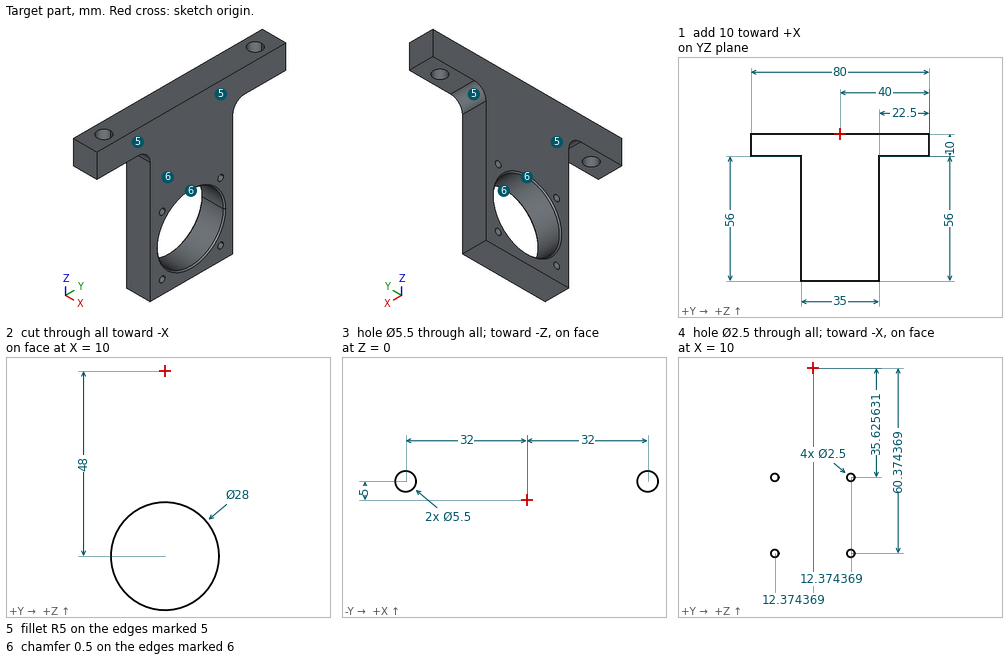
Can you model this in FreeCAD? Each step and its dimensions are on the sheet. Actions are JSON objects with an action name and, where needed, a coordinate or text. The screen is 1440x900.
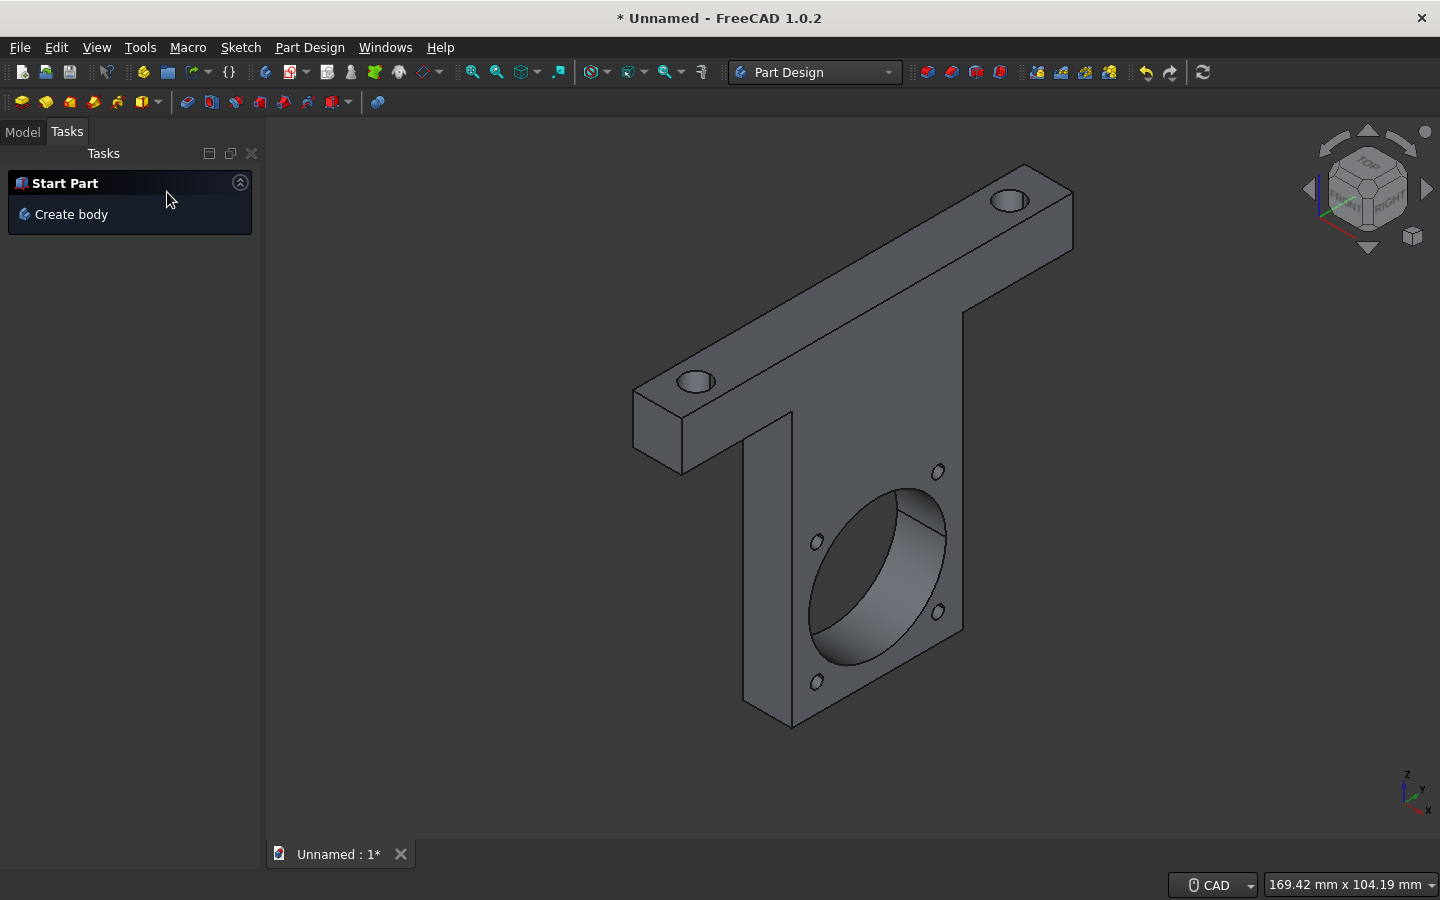
{"action": "key", "text": "2"}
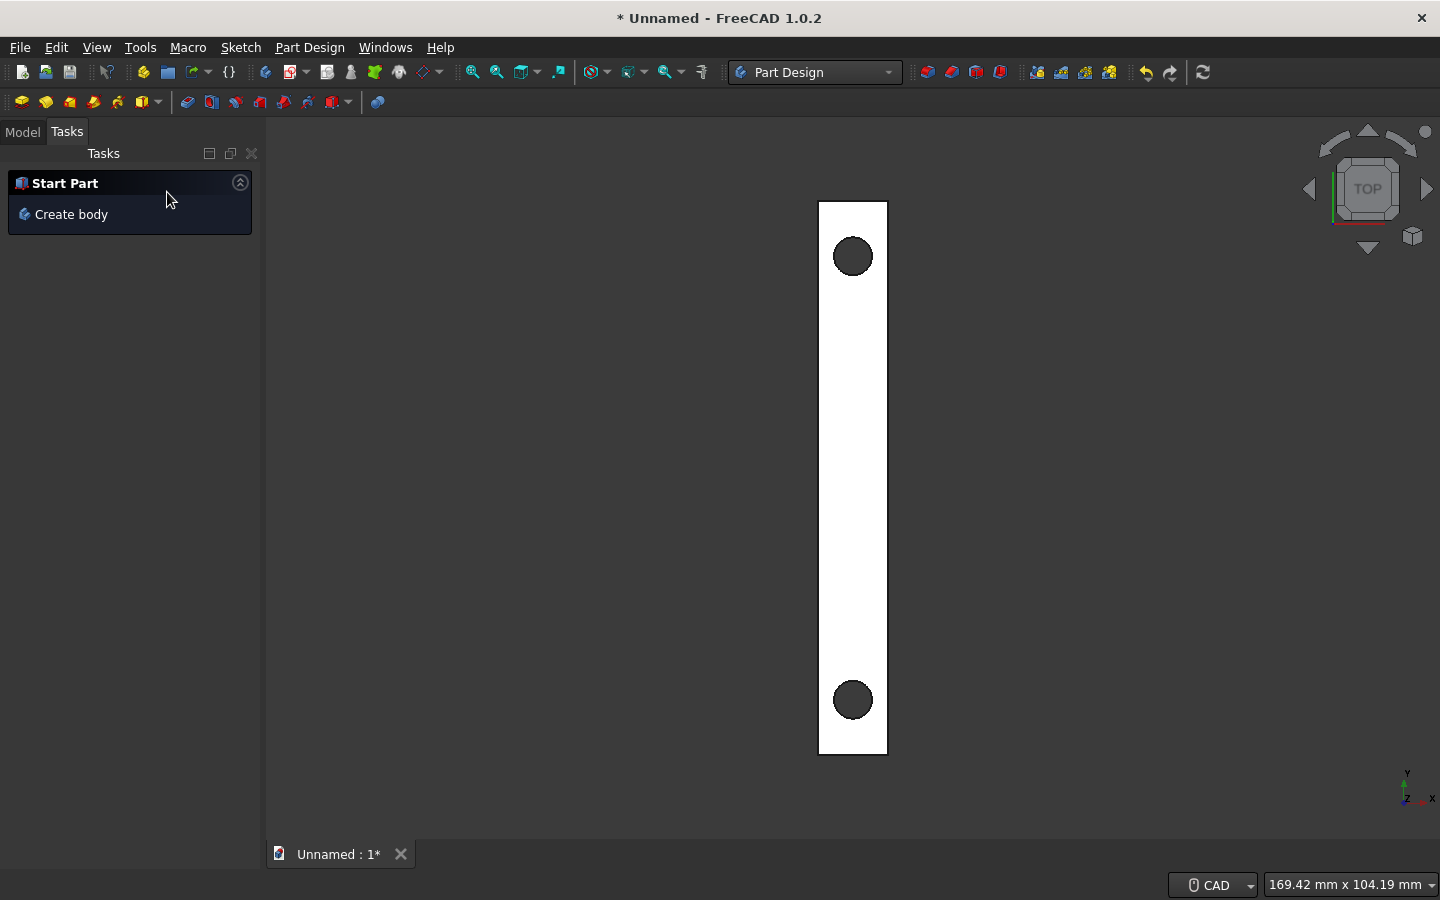
{"action": "key", "text": "1"}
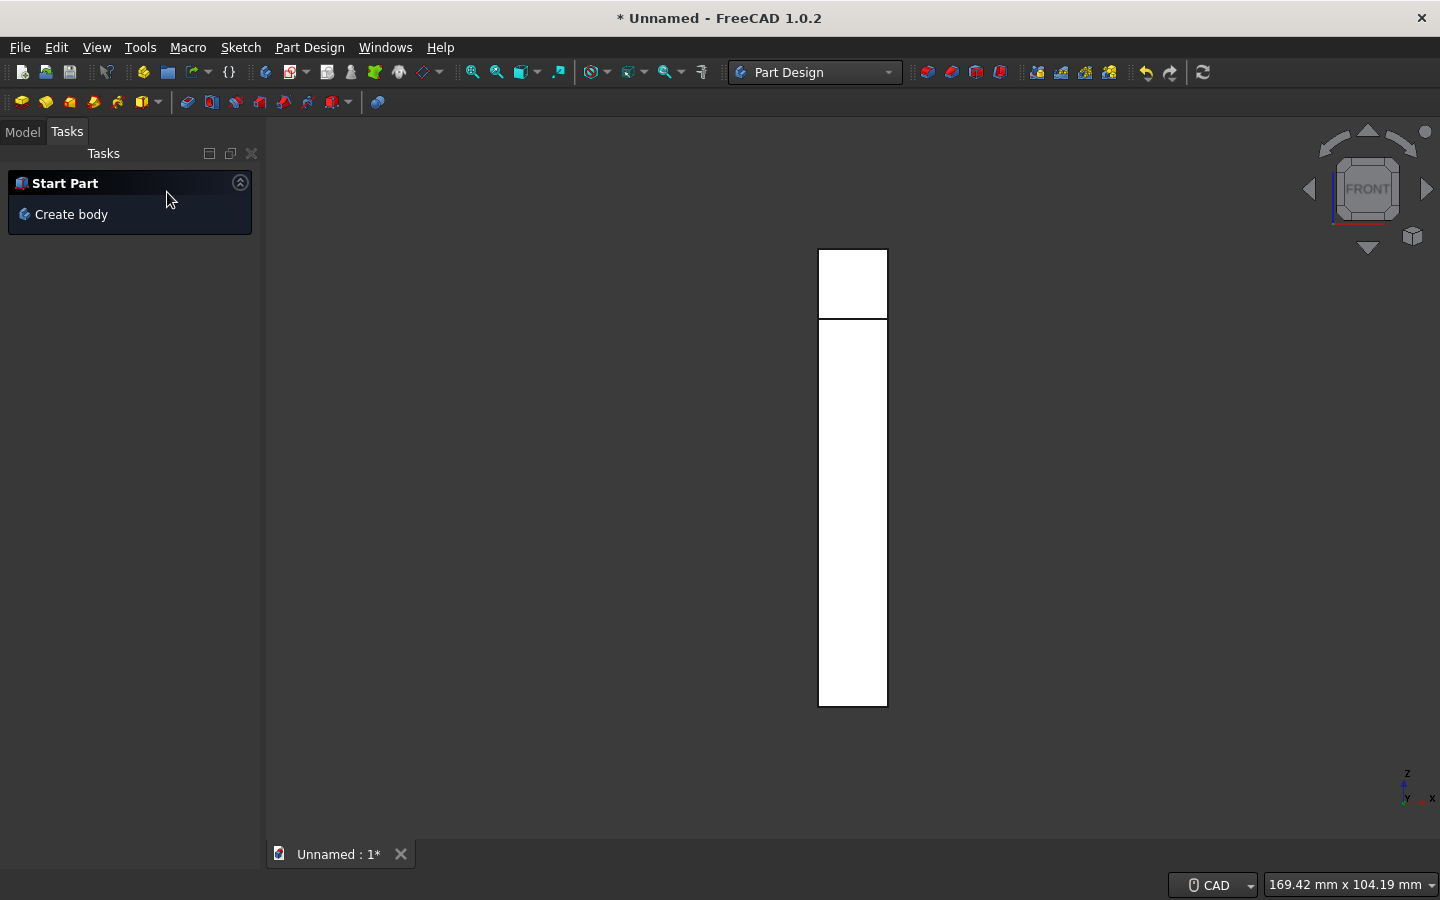
{"action": "key", "text": "3"}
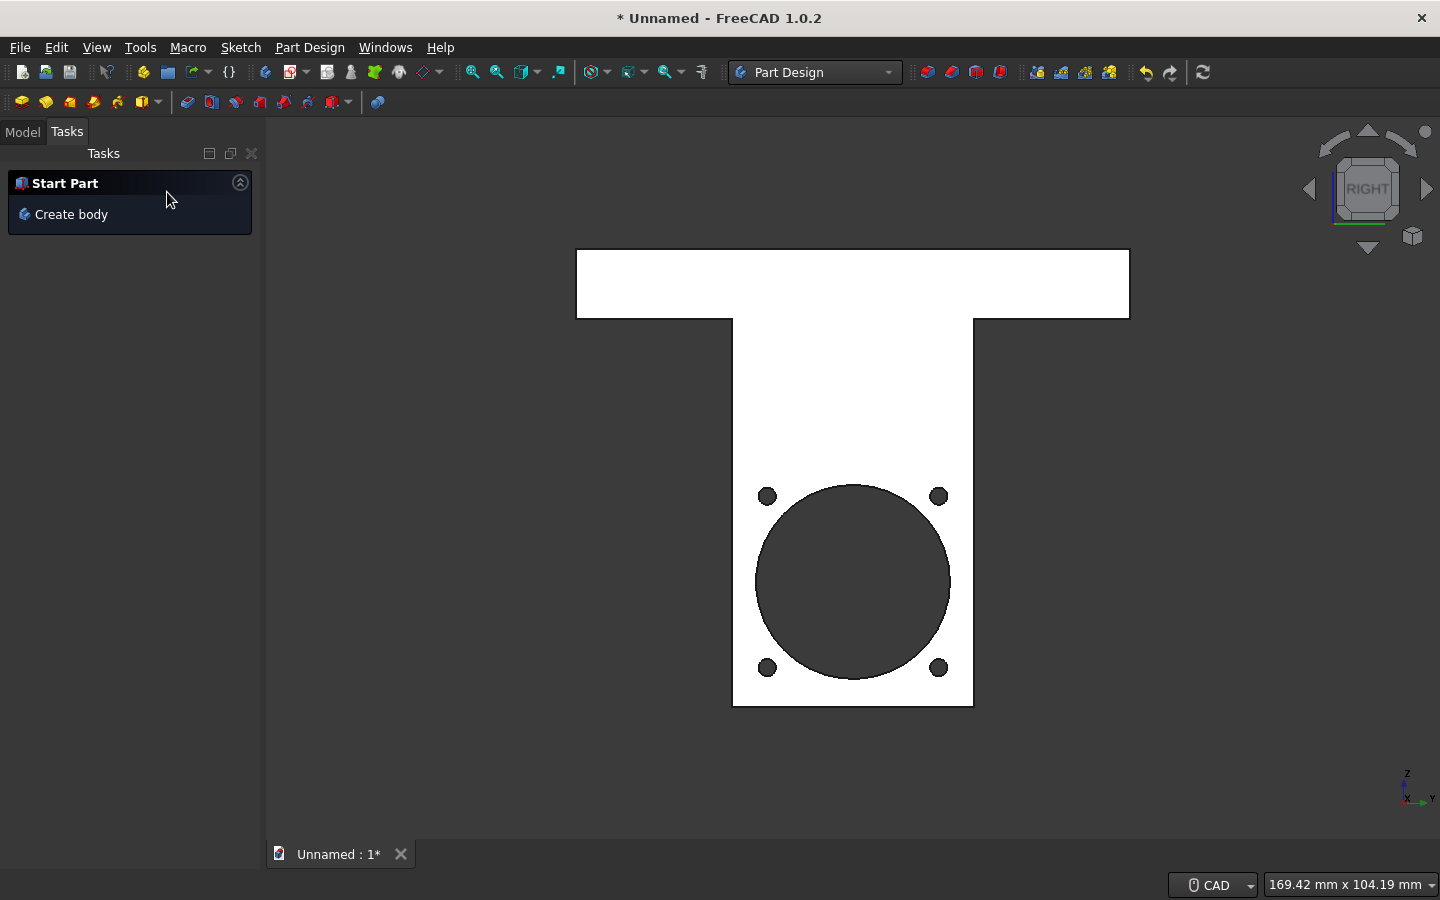
{"action": "key", "text": "5"}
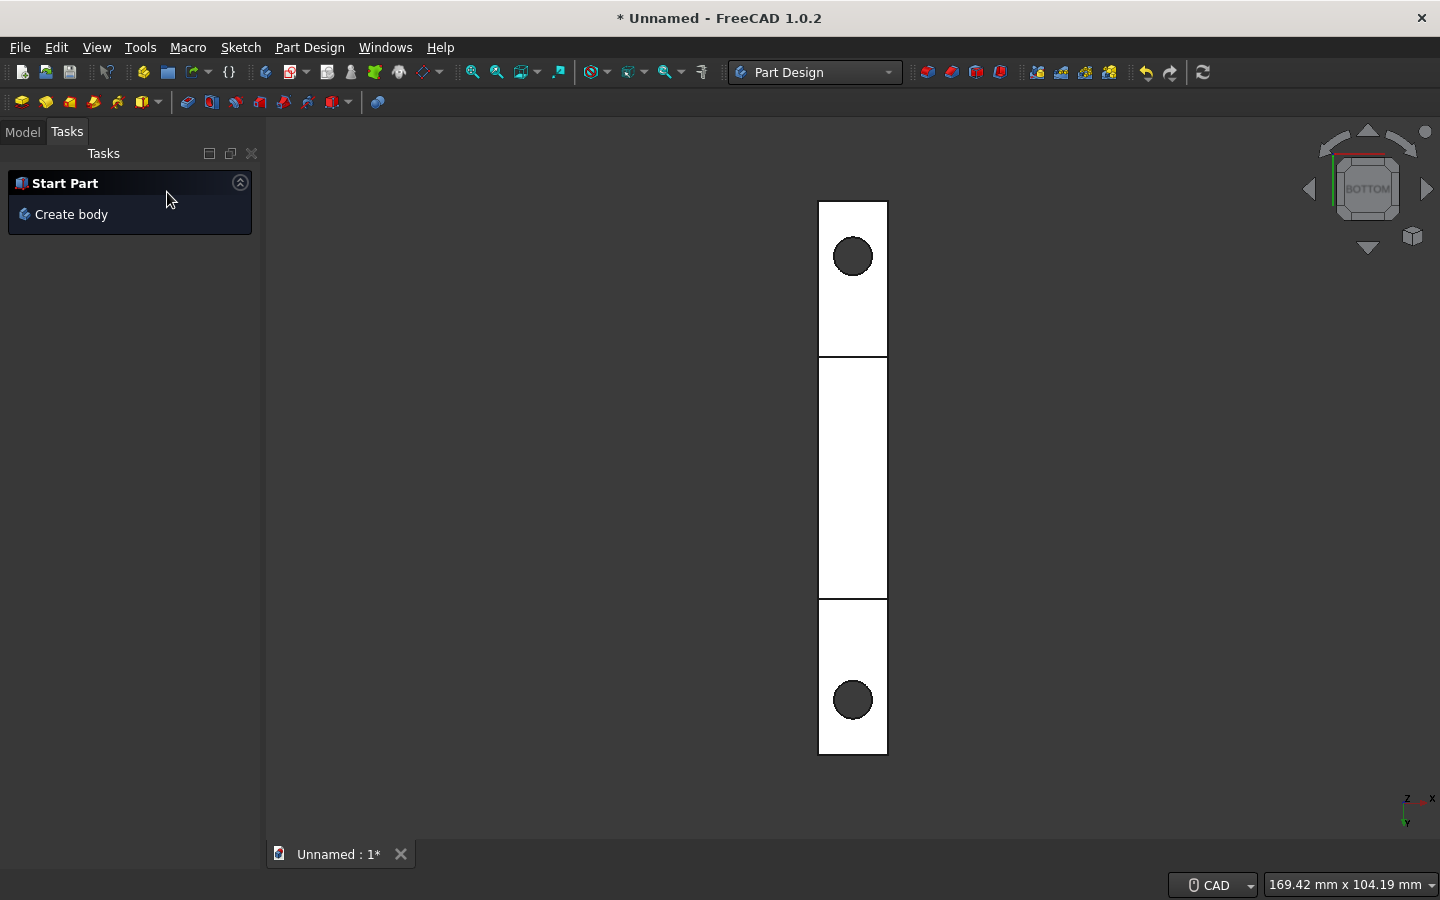
{"action": "key", "text": "4"}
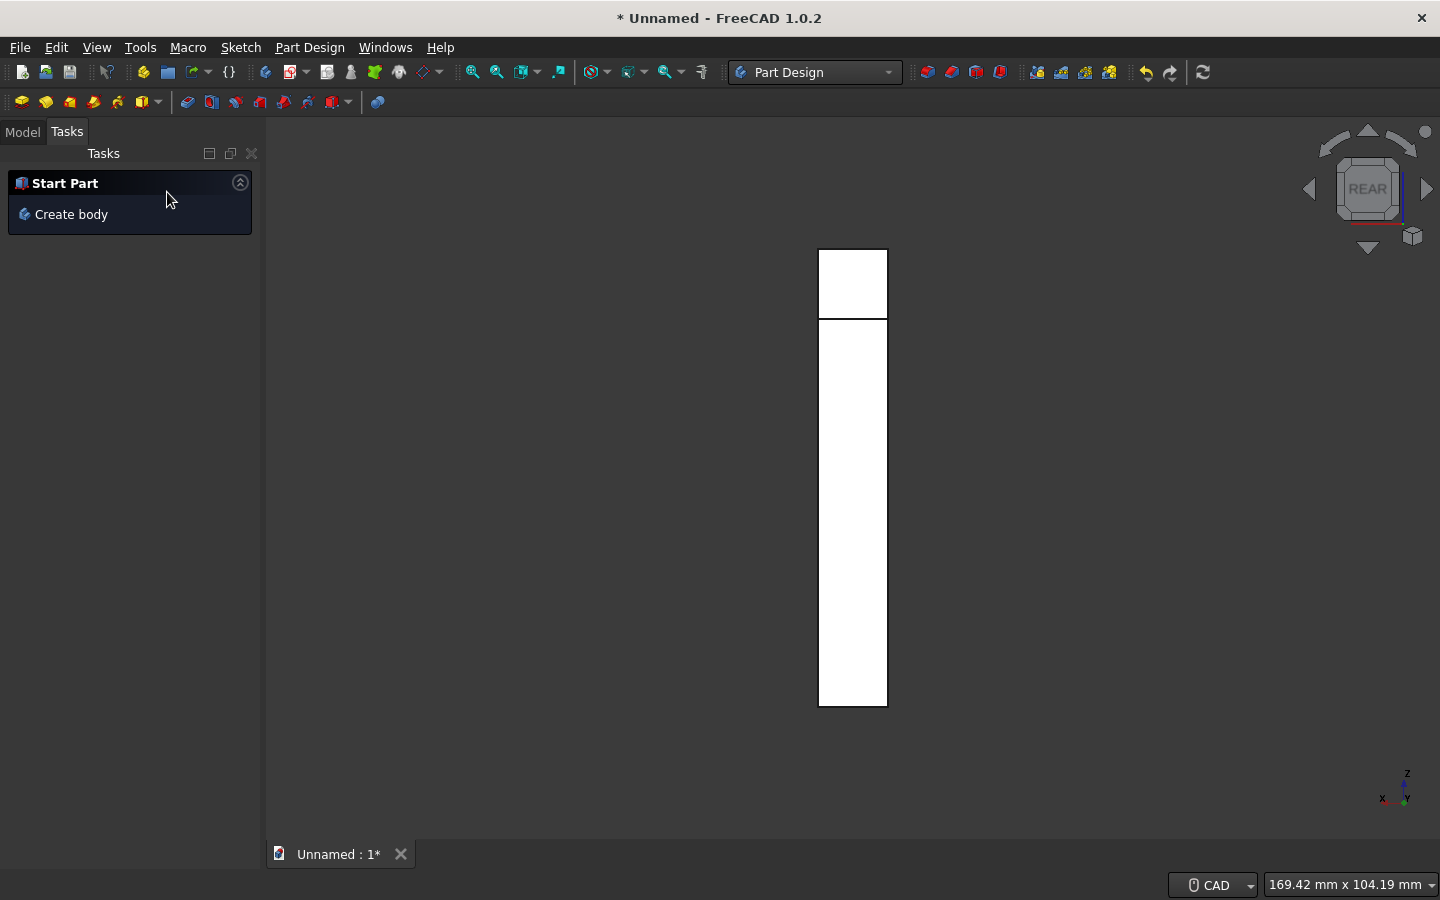
{"action": "key", "text": "6"}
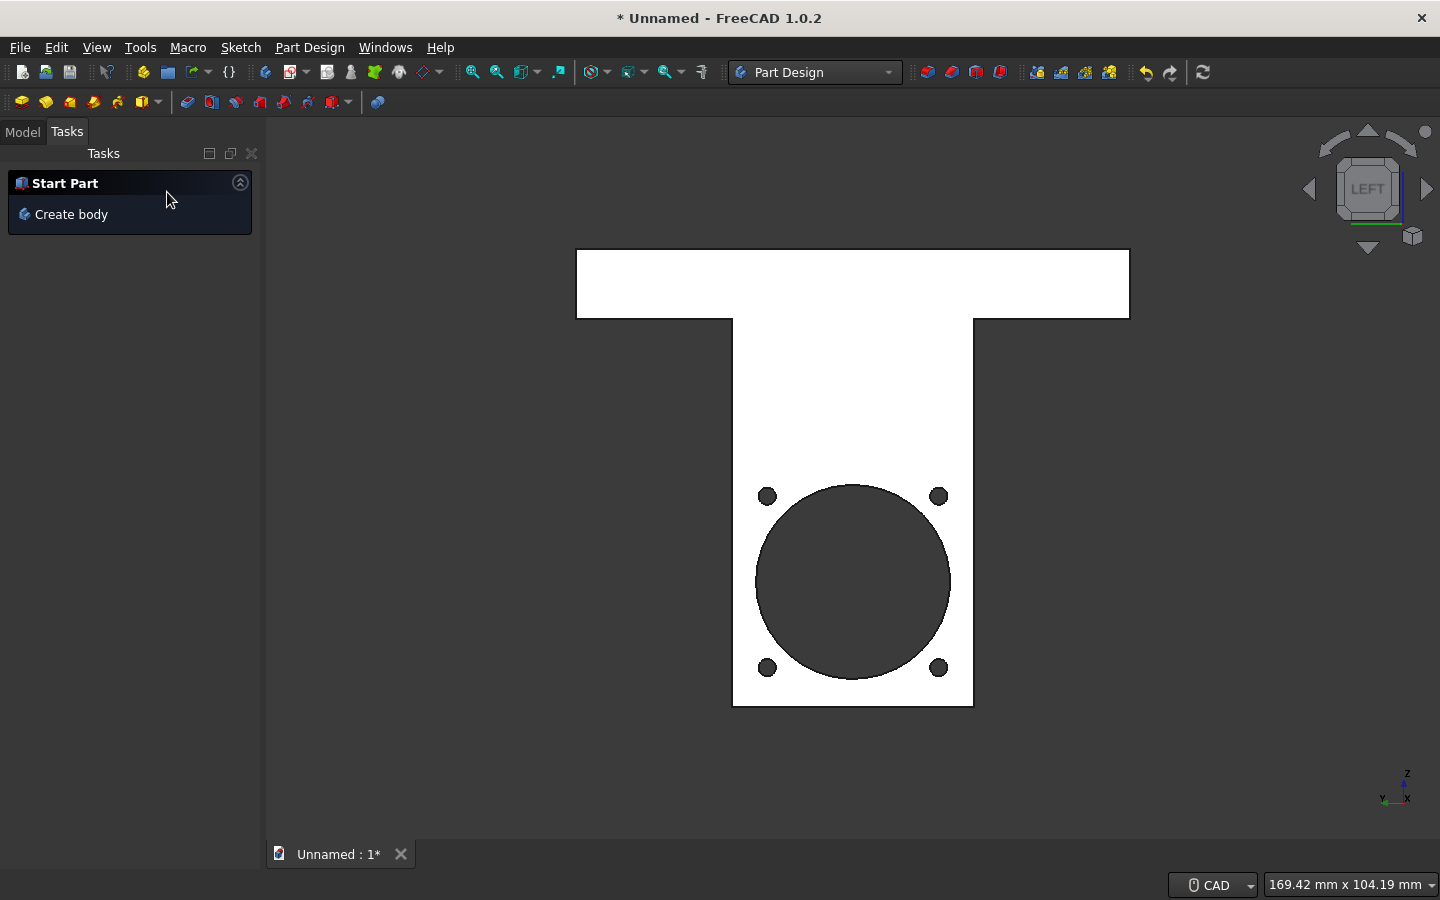
{"action": "key", "text": "v 3"}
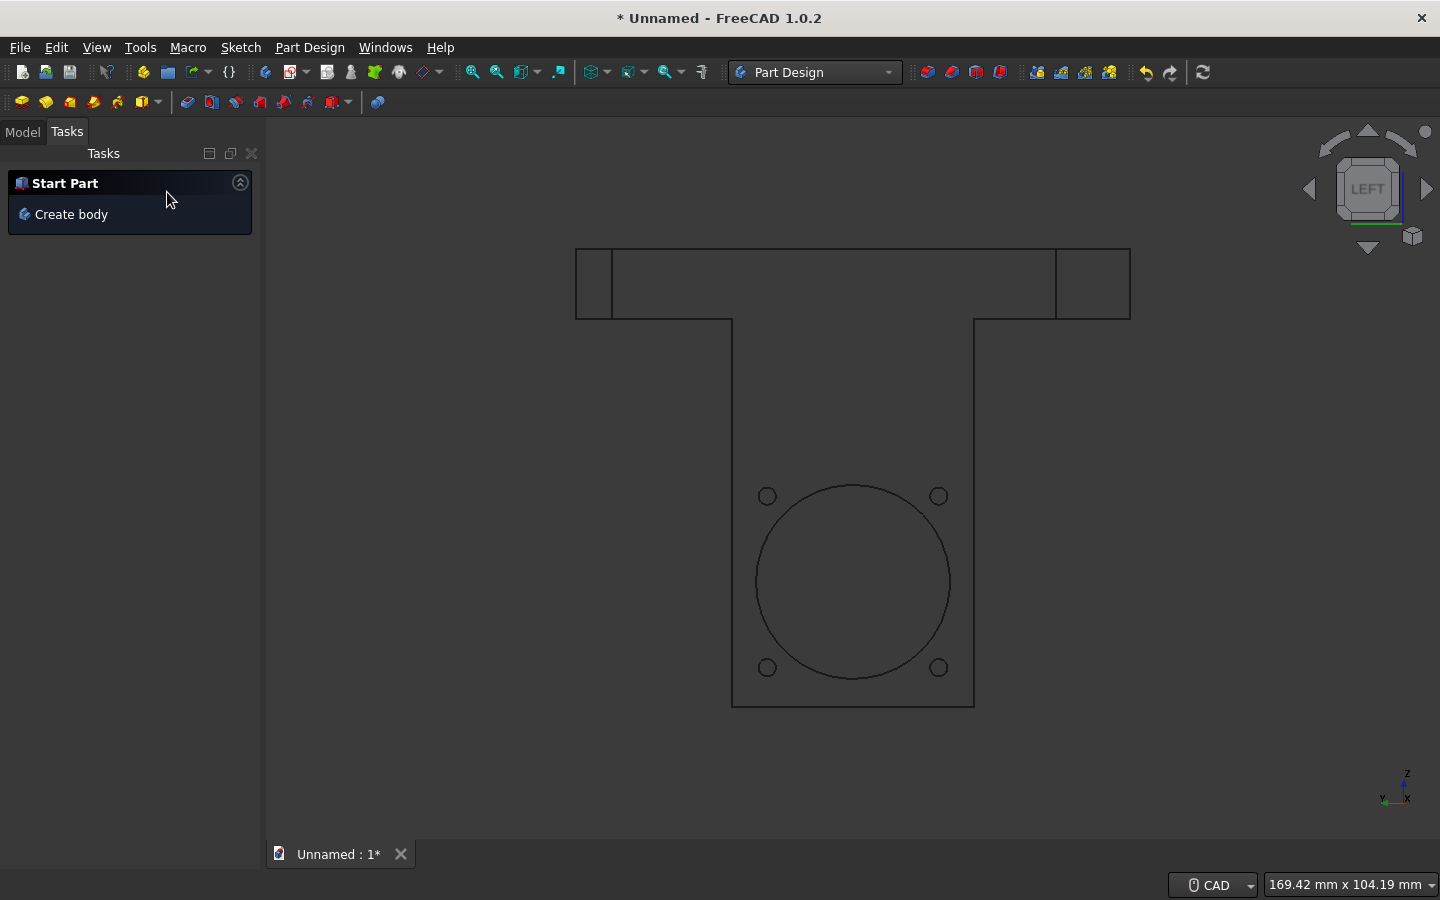
{"action": "key", "text": "0"}